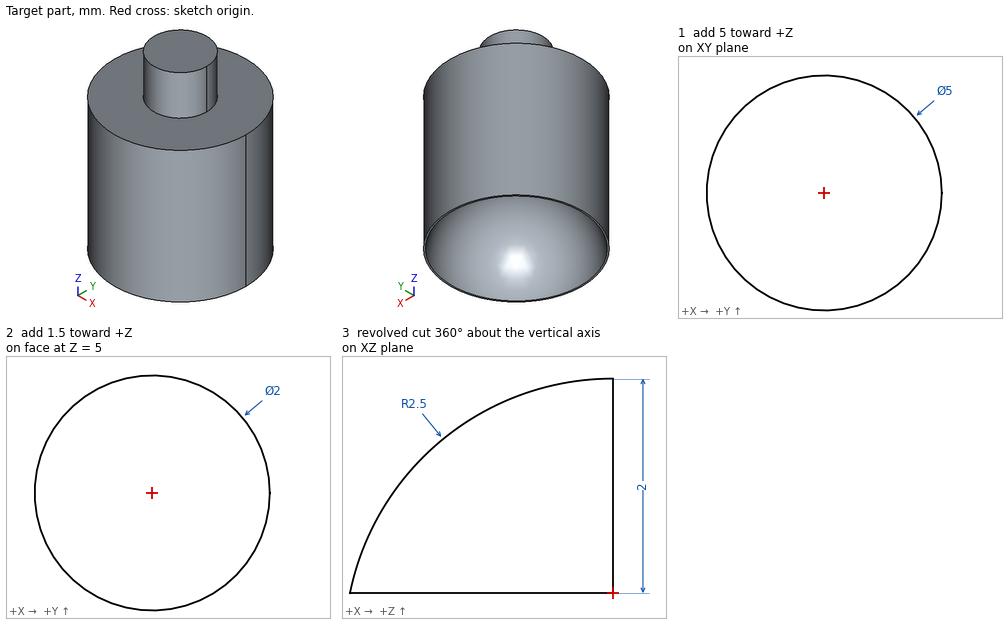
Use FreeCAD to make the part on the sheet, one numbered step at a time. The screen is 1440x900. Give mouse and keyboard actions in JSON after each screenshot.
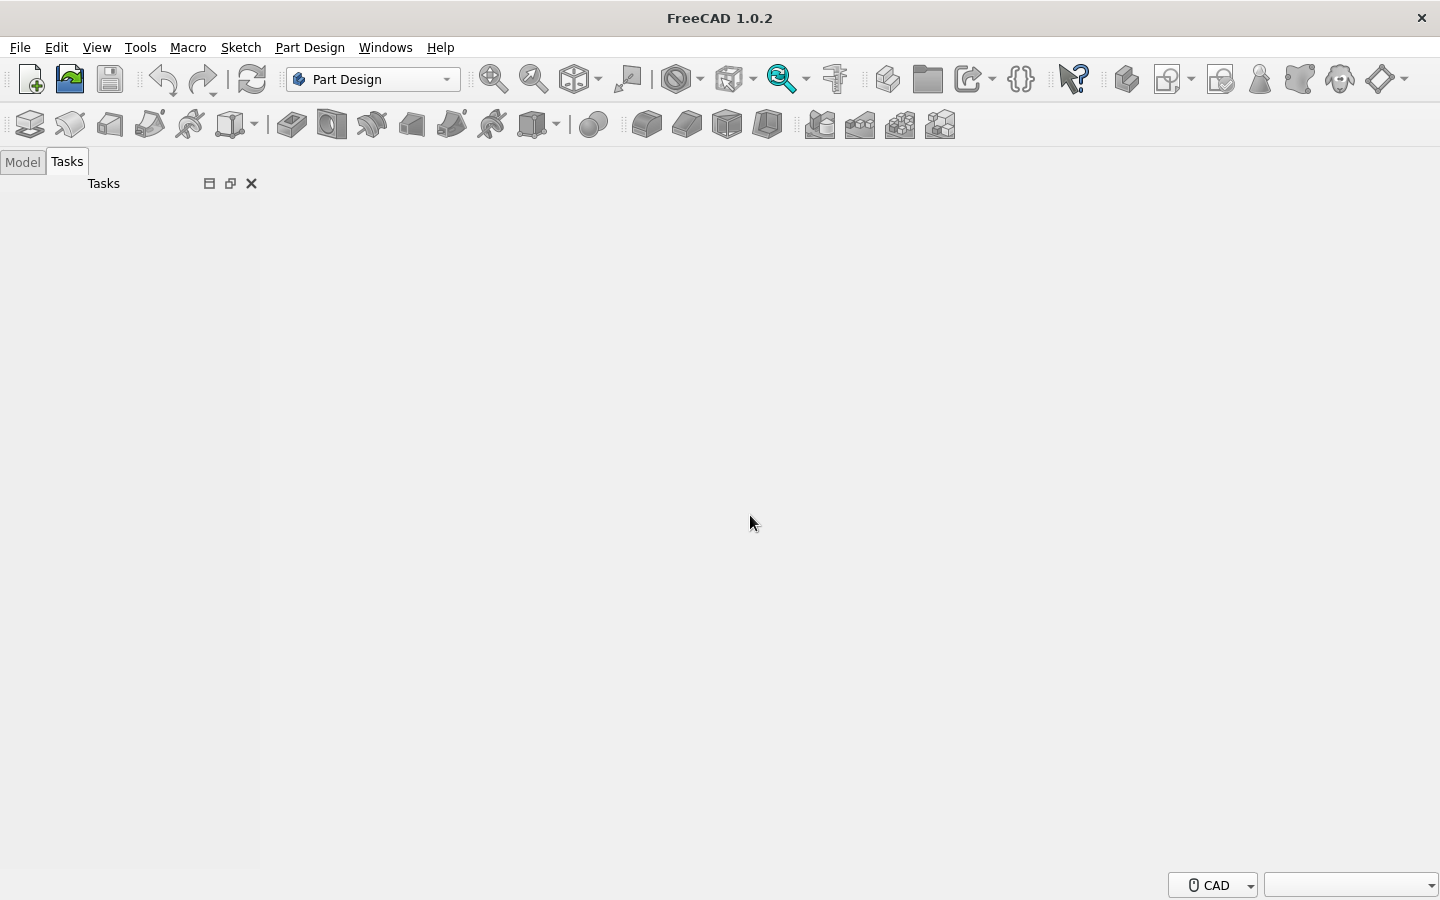
{"action": "left_click", "coordinate": [30, 80]}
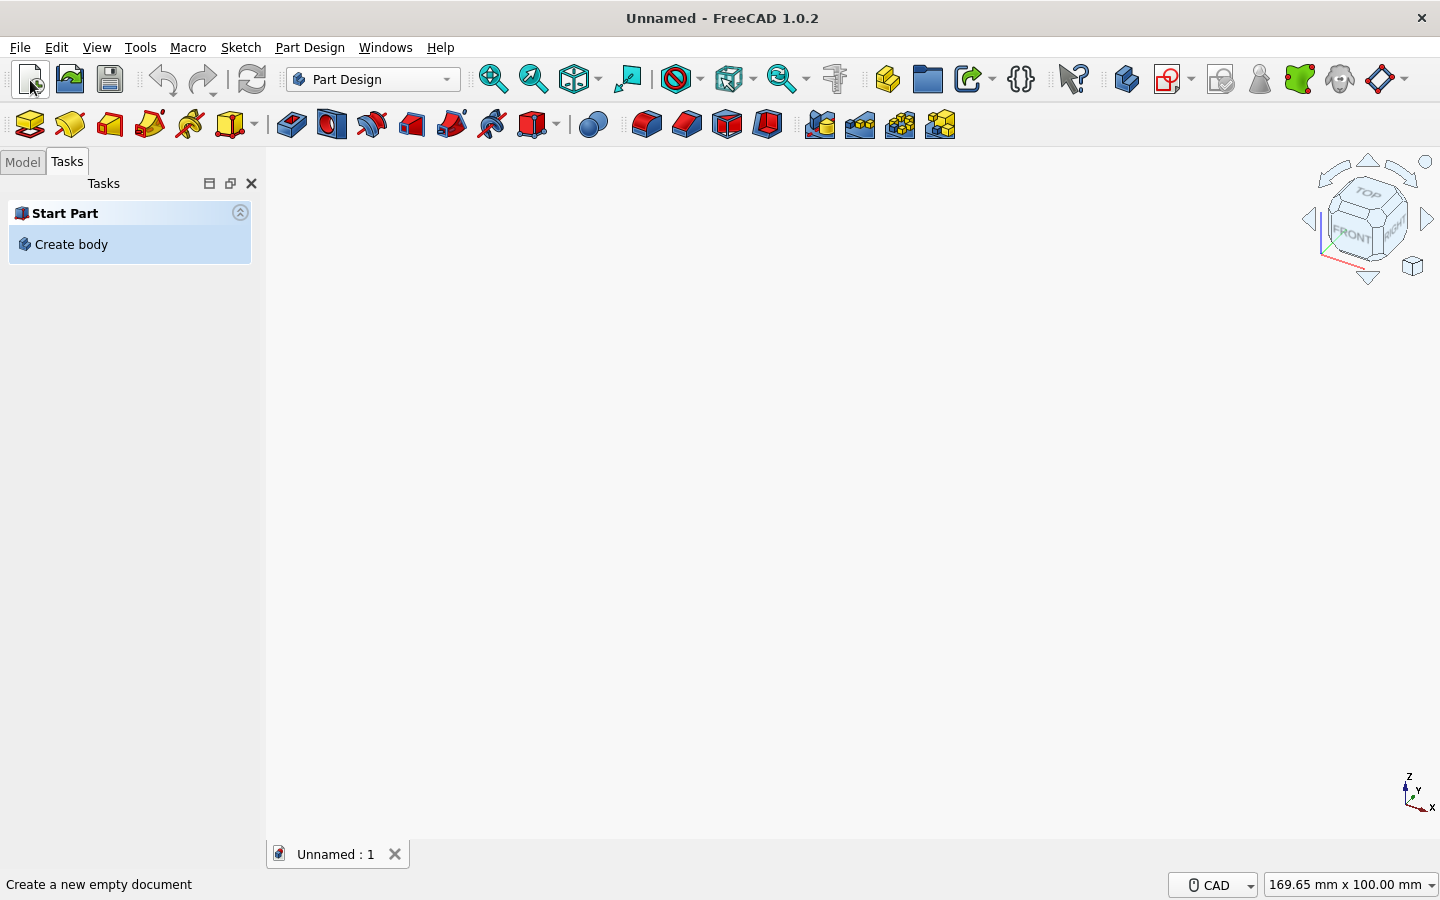
{"action": "left_click", "coordinate": [1168, 80]}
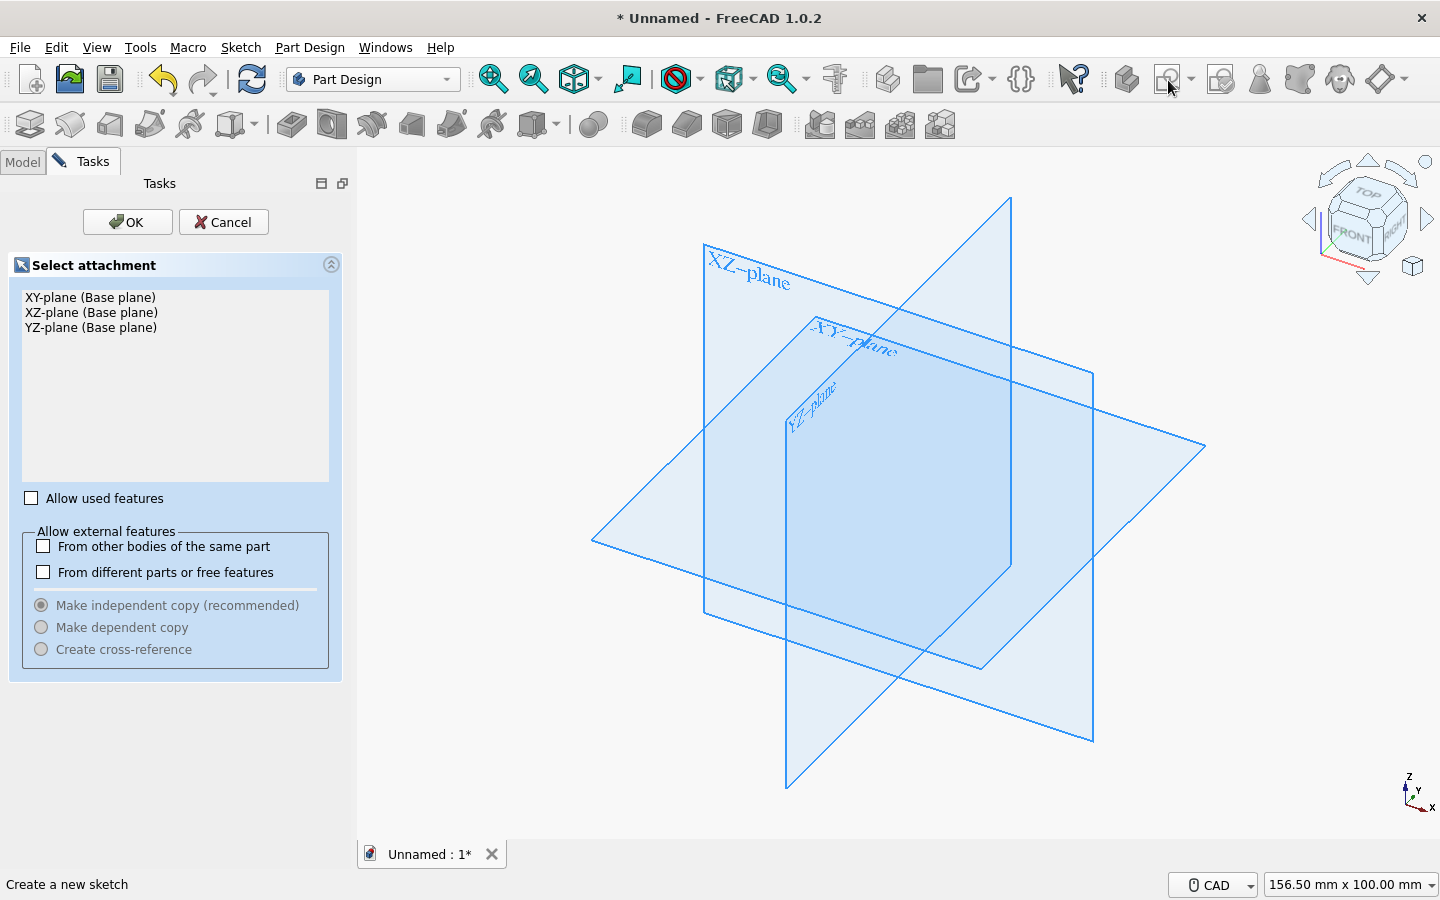
{"action": "left_click", "coordinate": [82, 298]}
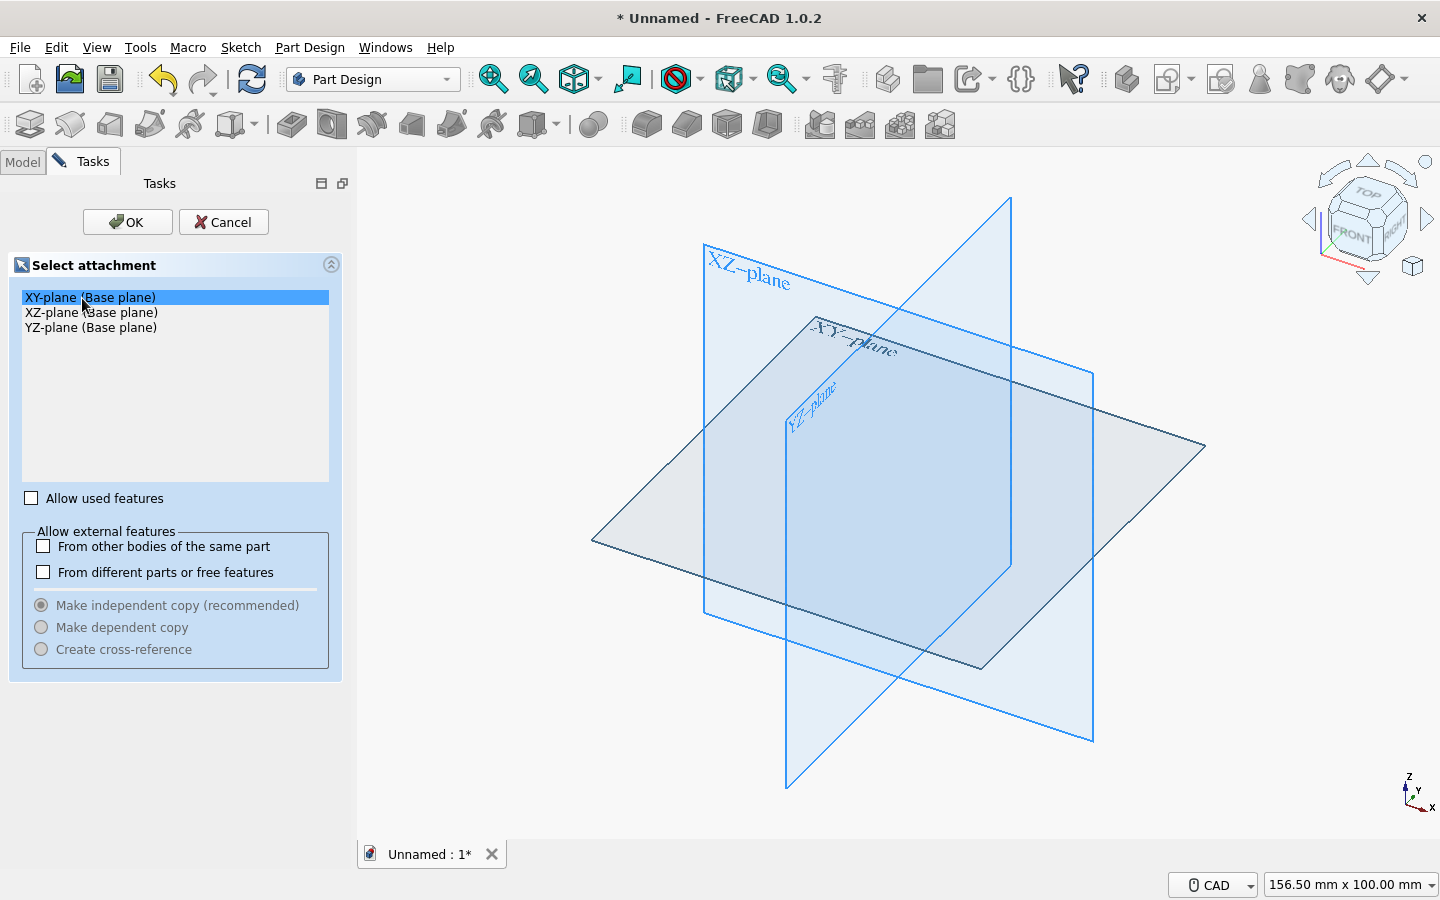
{"action": "left_click", "coordinate": [128, 222]}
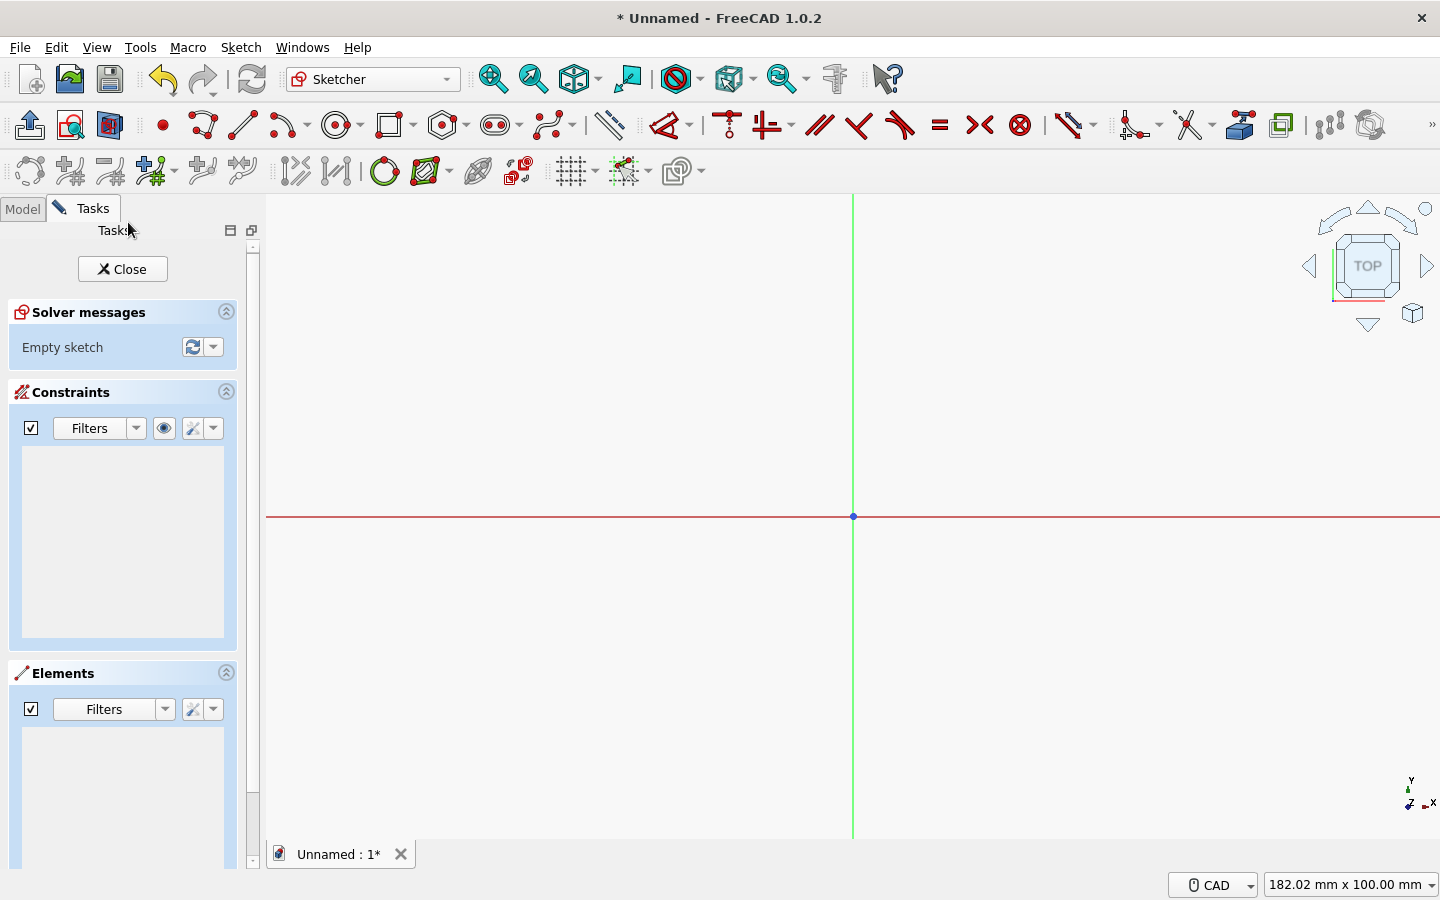
{"action": "scroll", "coordinate": [858, 516], "scroll_direction": "up", "scroll_amount": 13}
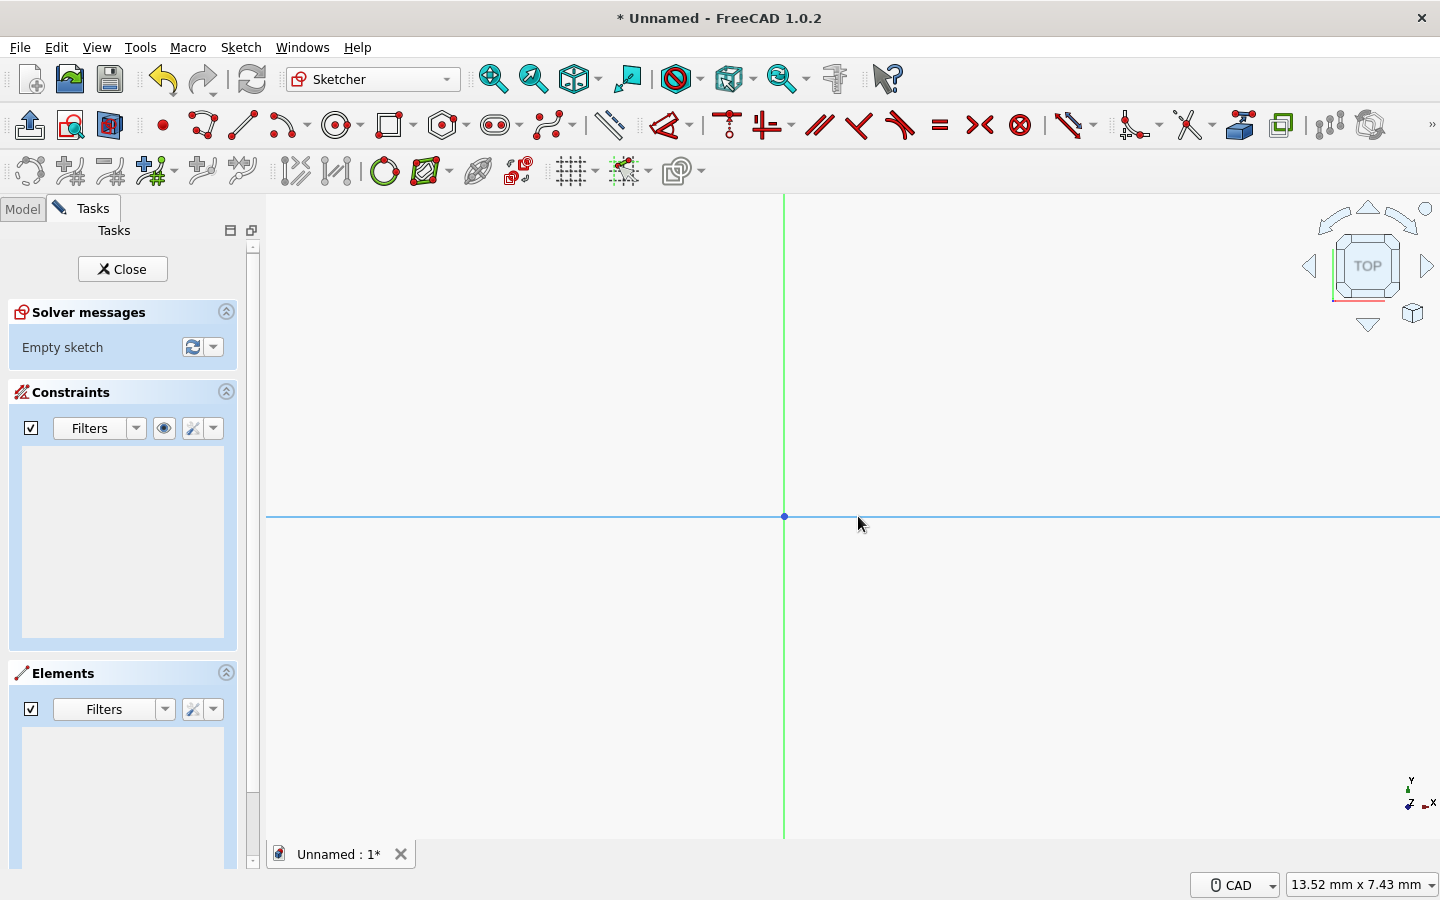
{"action": "left_click", "coordinate": [336, 126]}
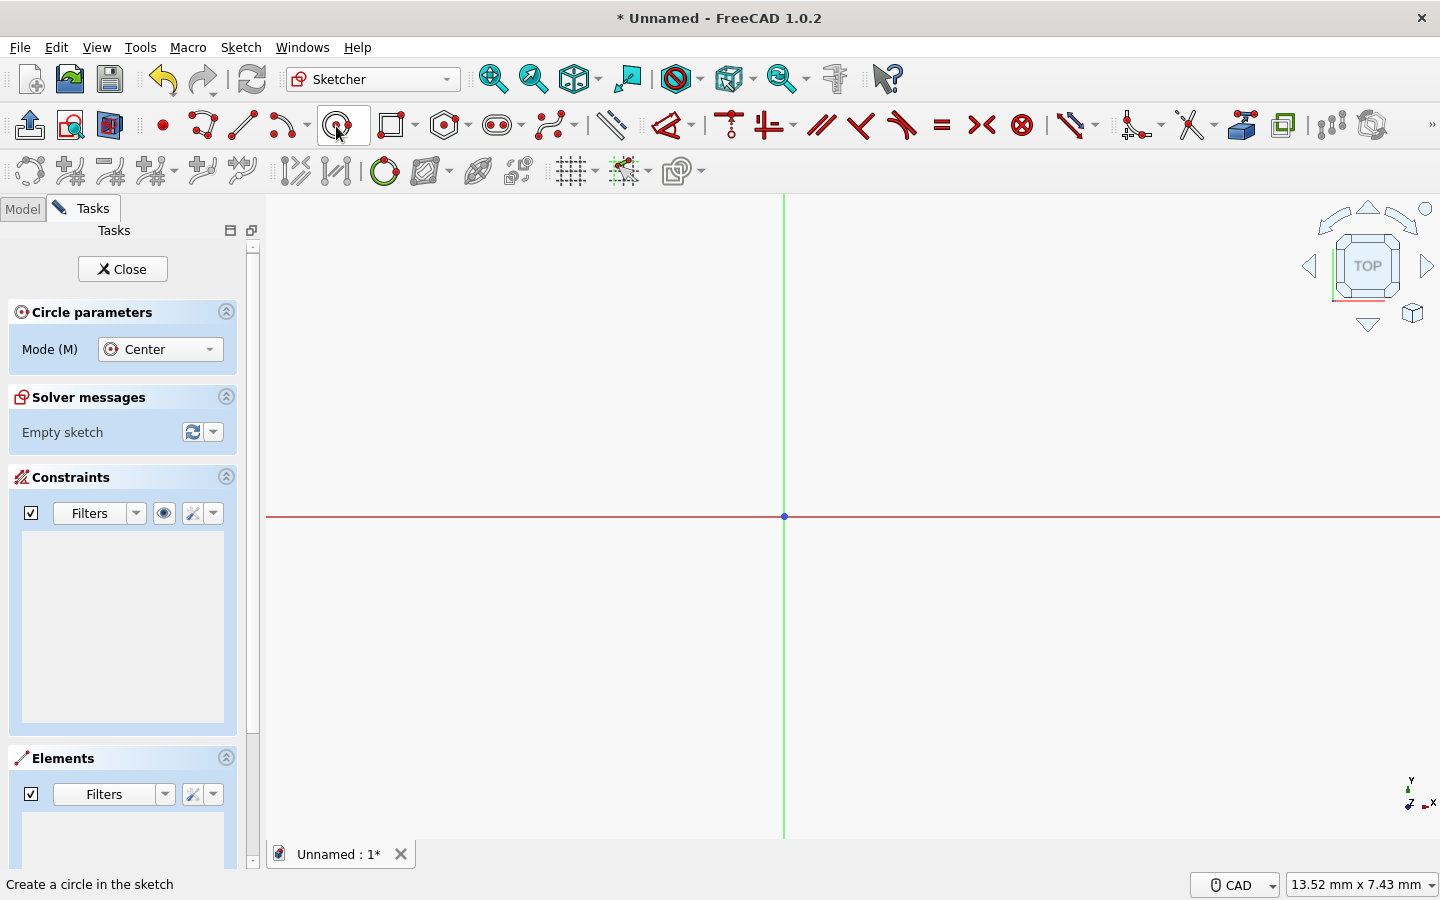
{"action": "left_click", "coordinate": [784, 516]}
{"action": "mouse_move", "coordinate": [938, 363]}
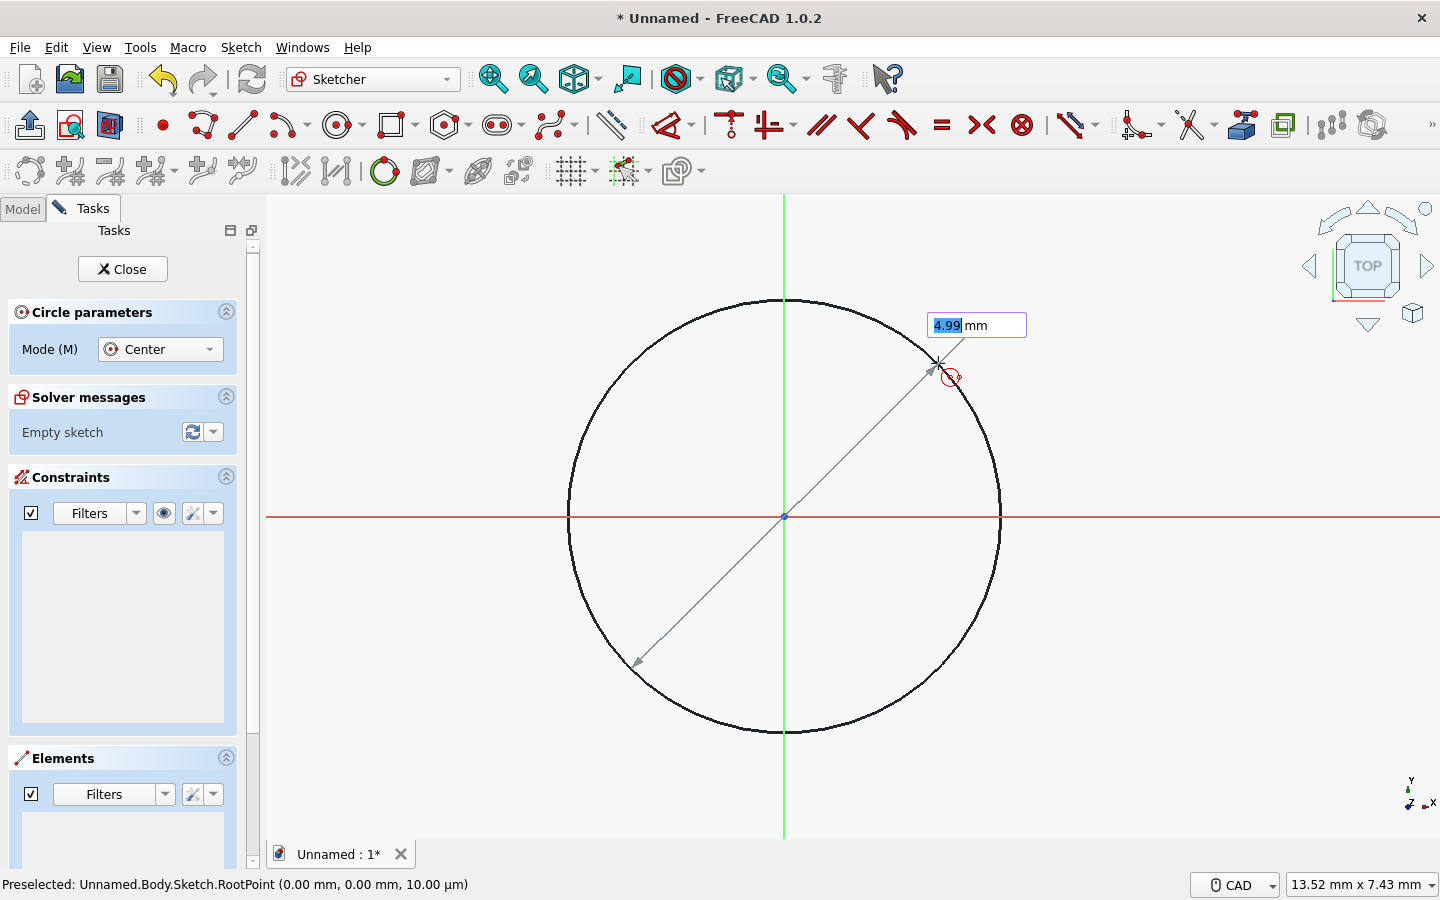
{"action": "type", "text": "5"}
{"action": "key", "text": "Return"}
{"action": "key", "text": "Escape"}